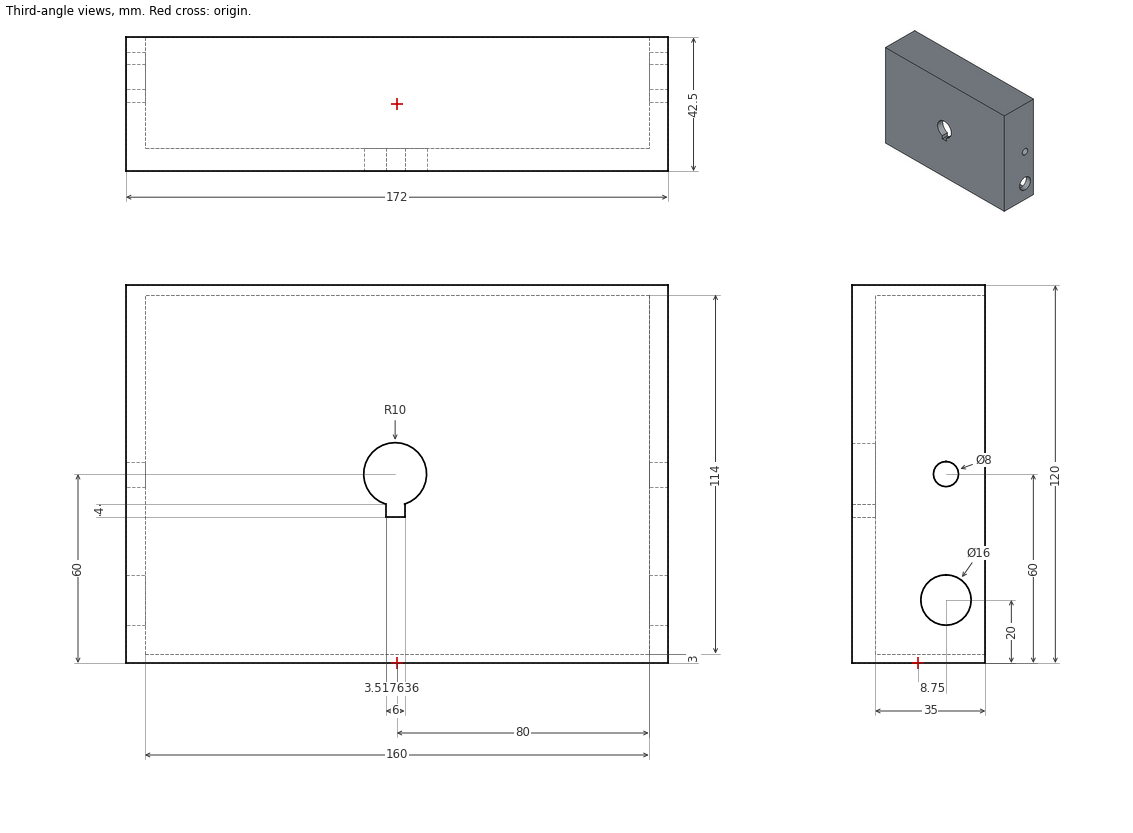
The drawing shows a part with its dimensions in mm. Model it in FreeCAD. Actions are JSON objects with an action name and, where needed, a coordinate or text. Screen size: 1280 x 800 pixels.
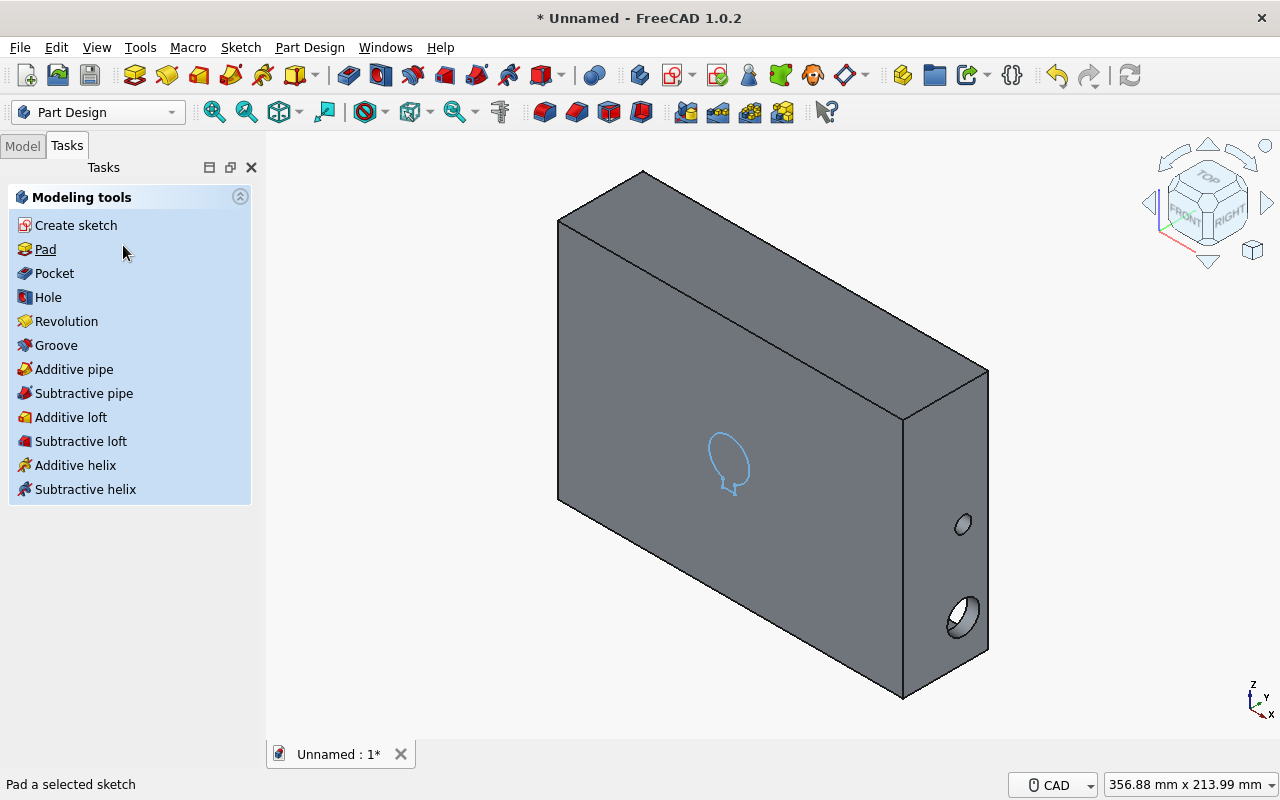
{"action": "left_click", "coordinate": [350, 76]}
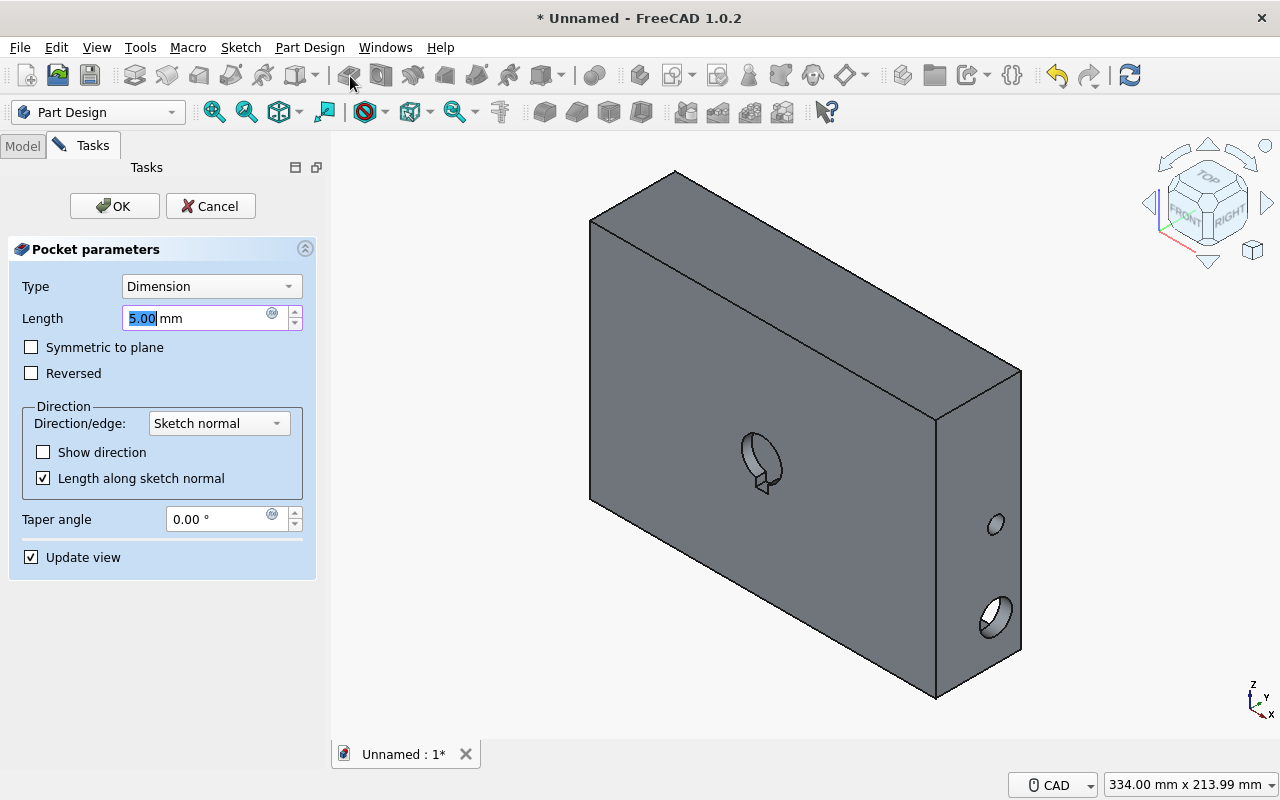
{"action": "left_click", "coordinate": [212, 286]}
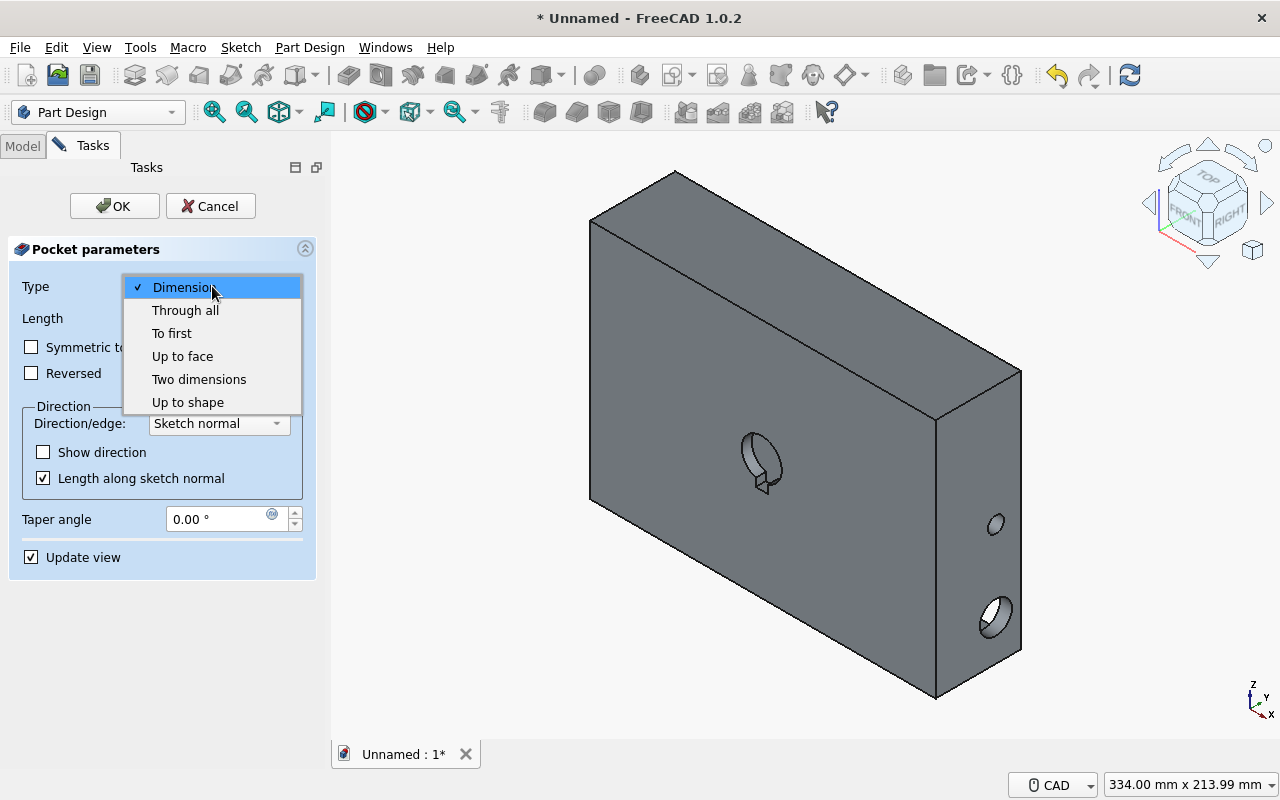
{"action": "left_click", "coordinate": [212, 310]}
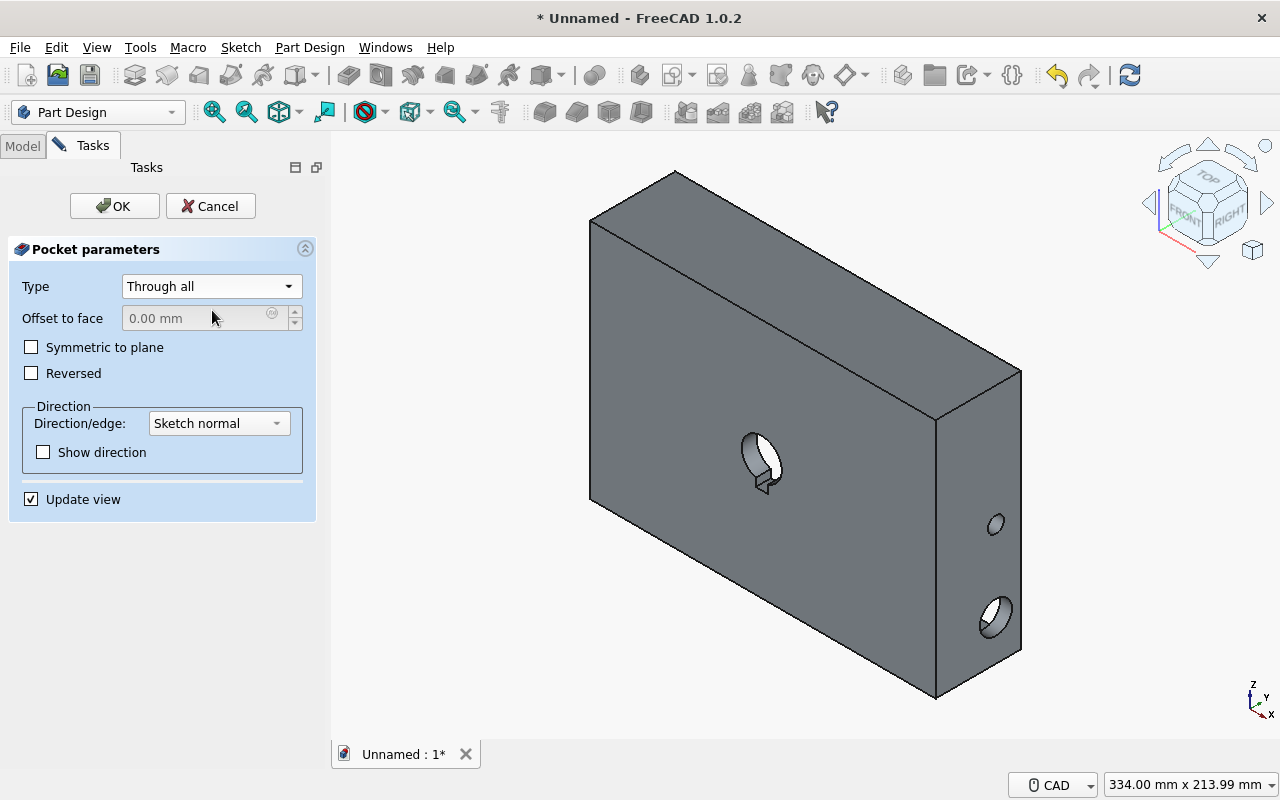
{"action": "left_click", "coordinate": [115, 206]}